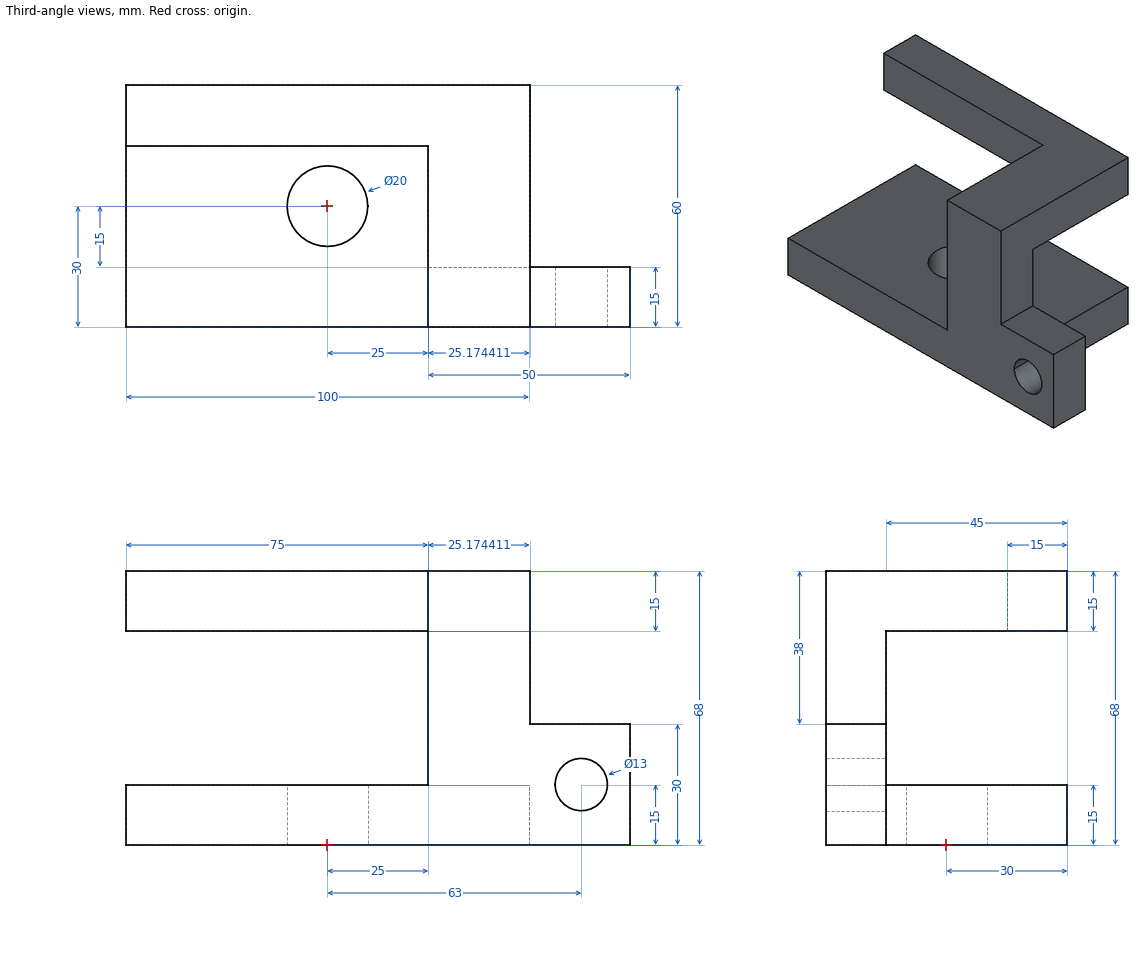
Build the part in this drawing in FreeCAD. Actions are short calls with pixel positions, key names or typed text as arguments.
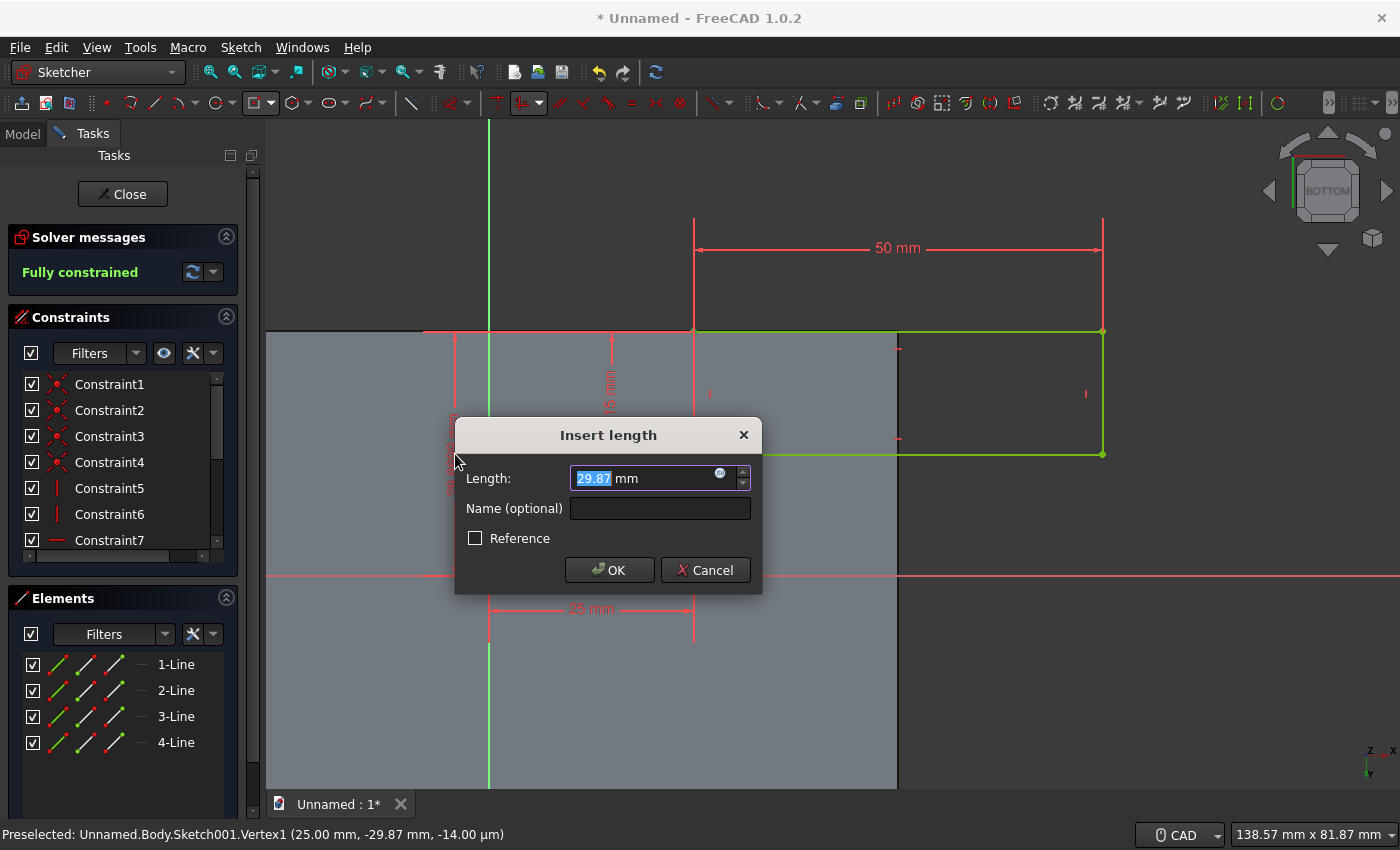
text(30)
key(Return)
key(Escape)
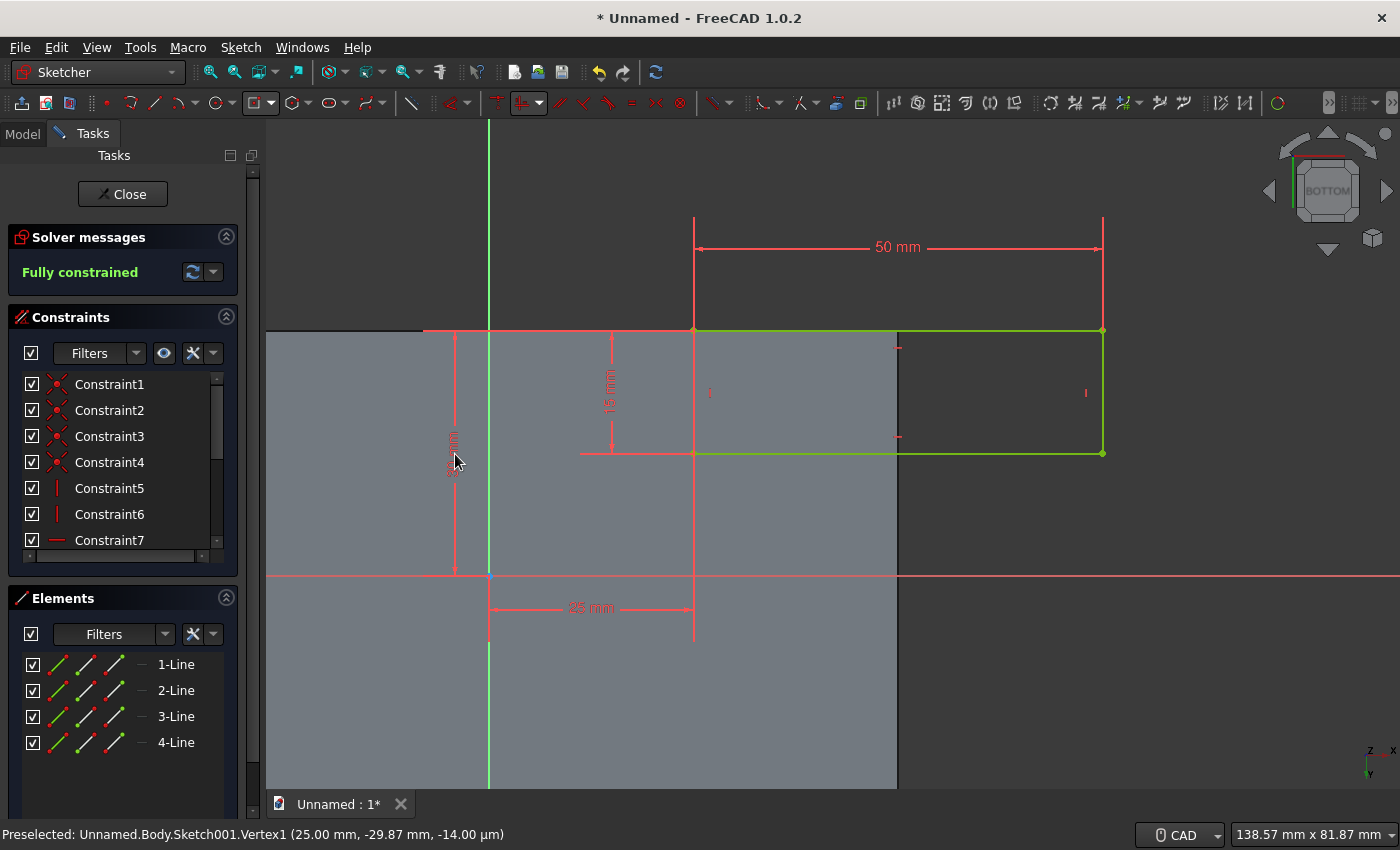
click(123, 194)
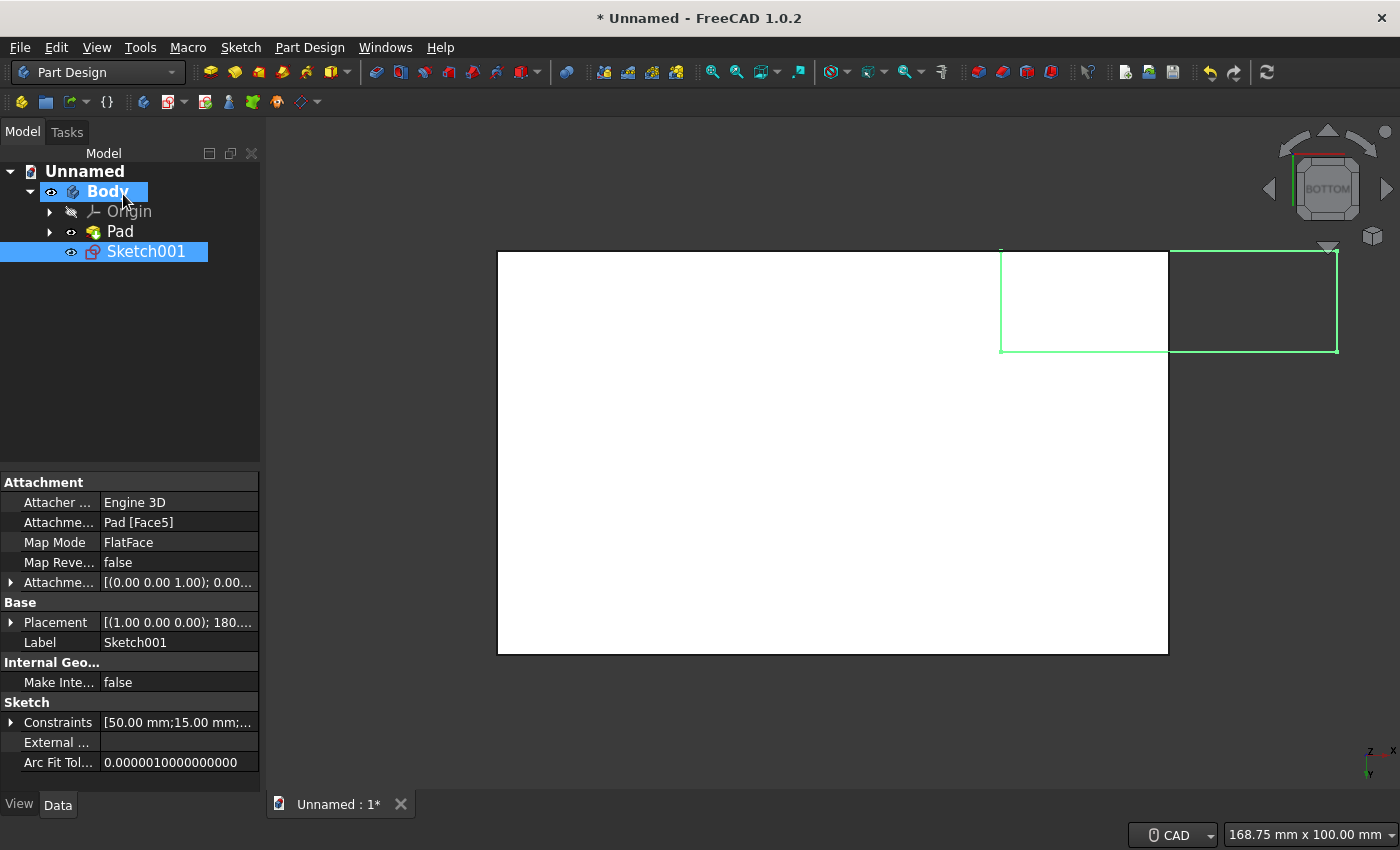
click(212, 72)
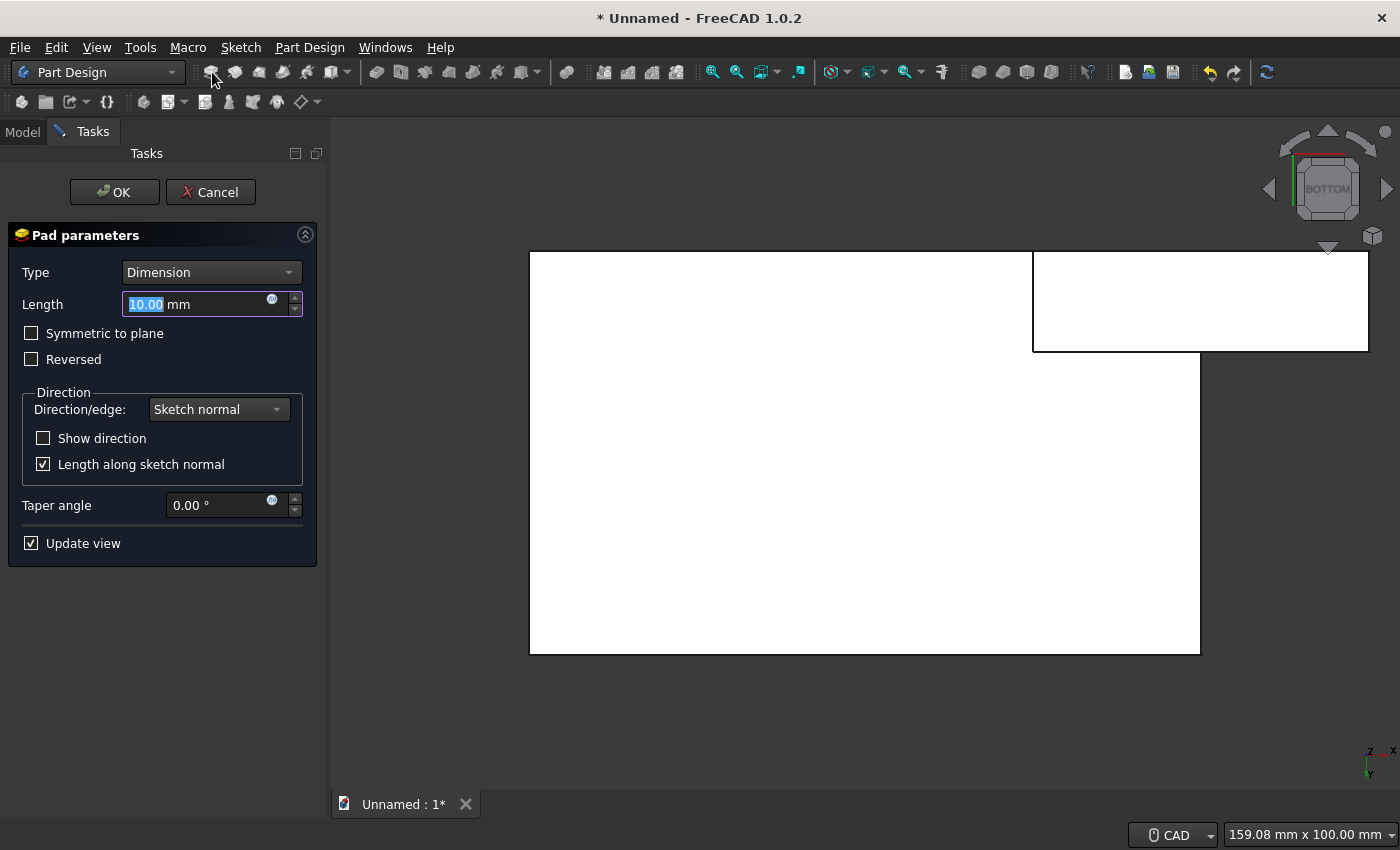
text(30)
key(Tab)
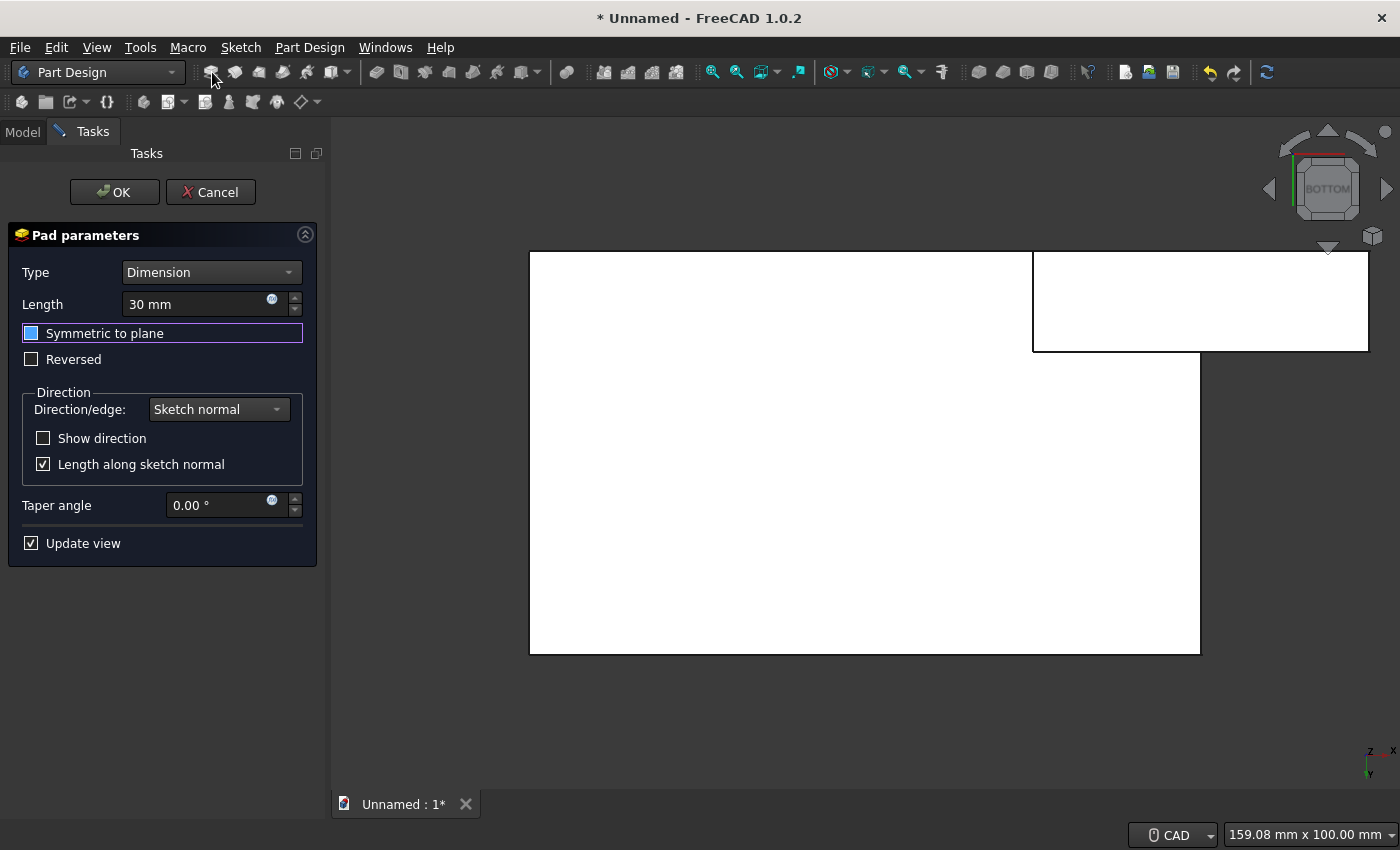
click(30, 359)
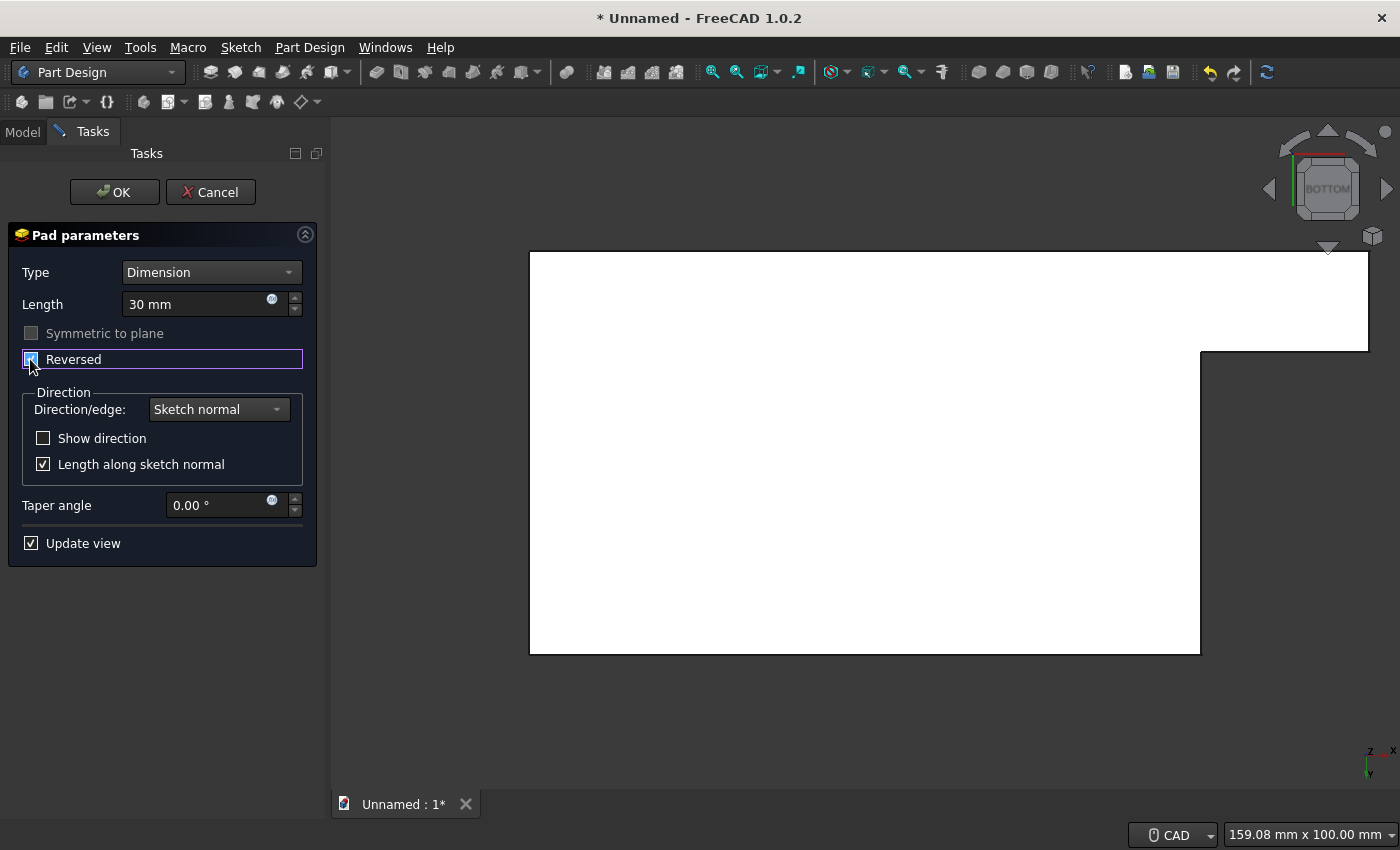
click(115, 192)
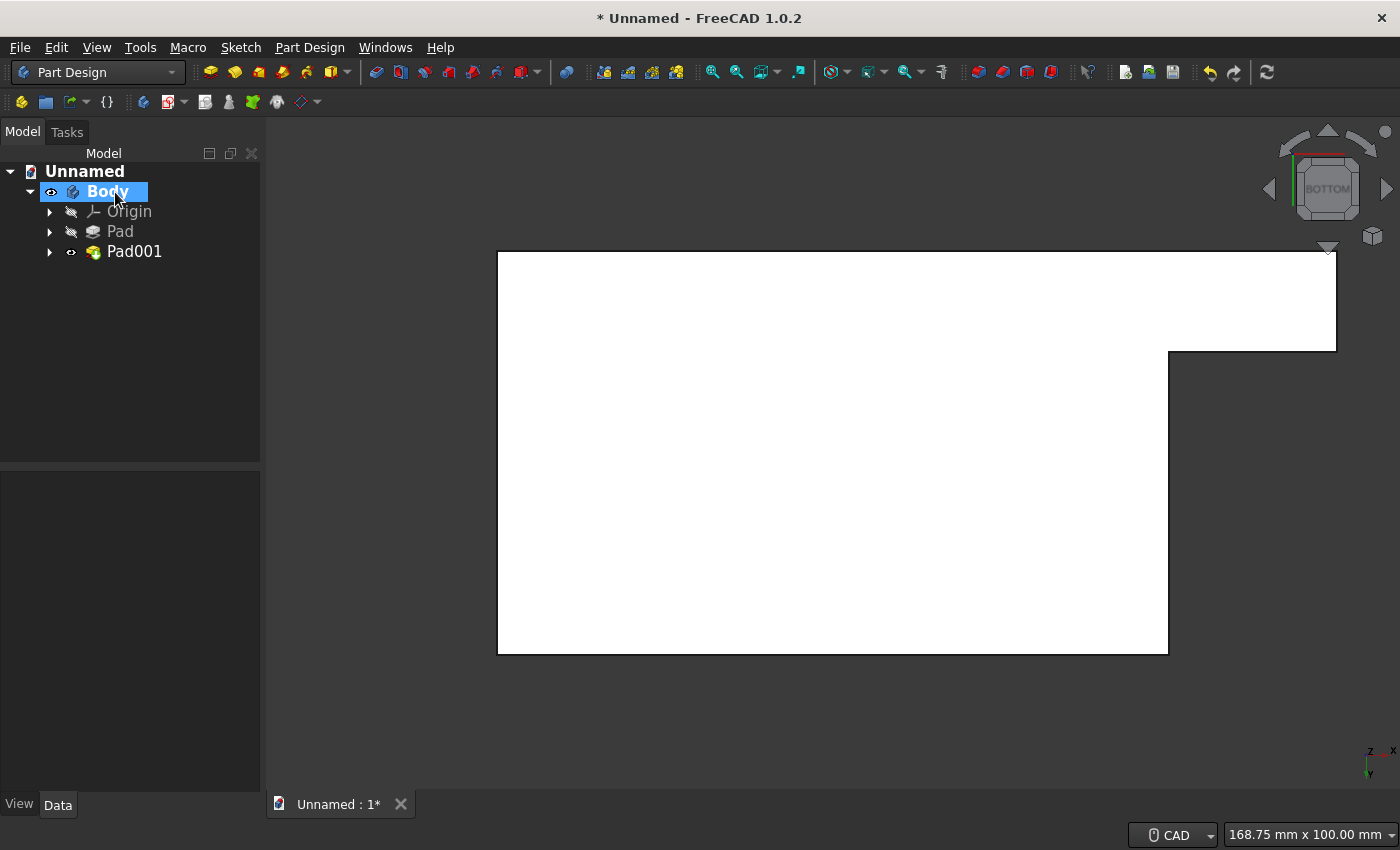
key(0)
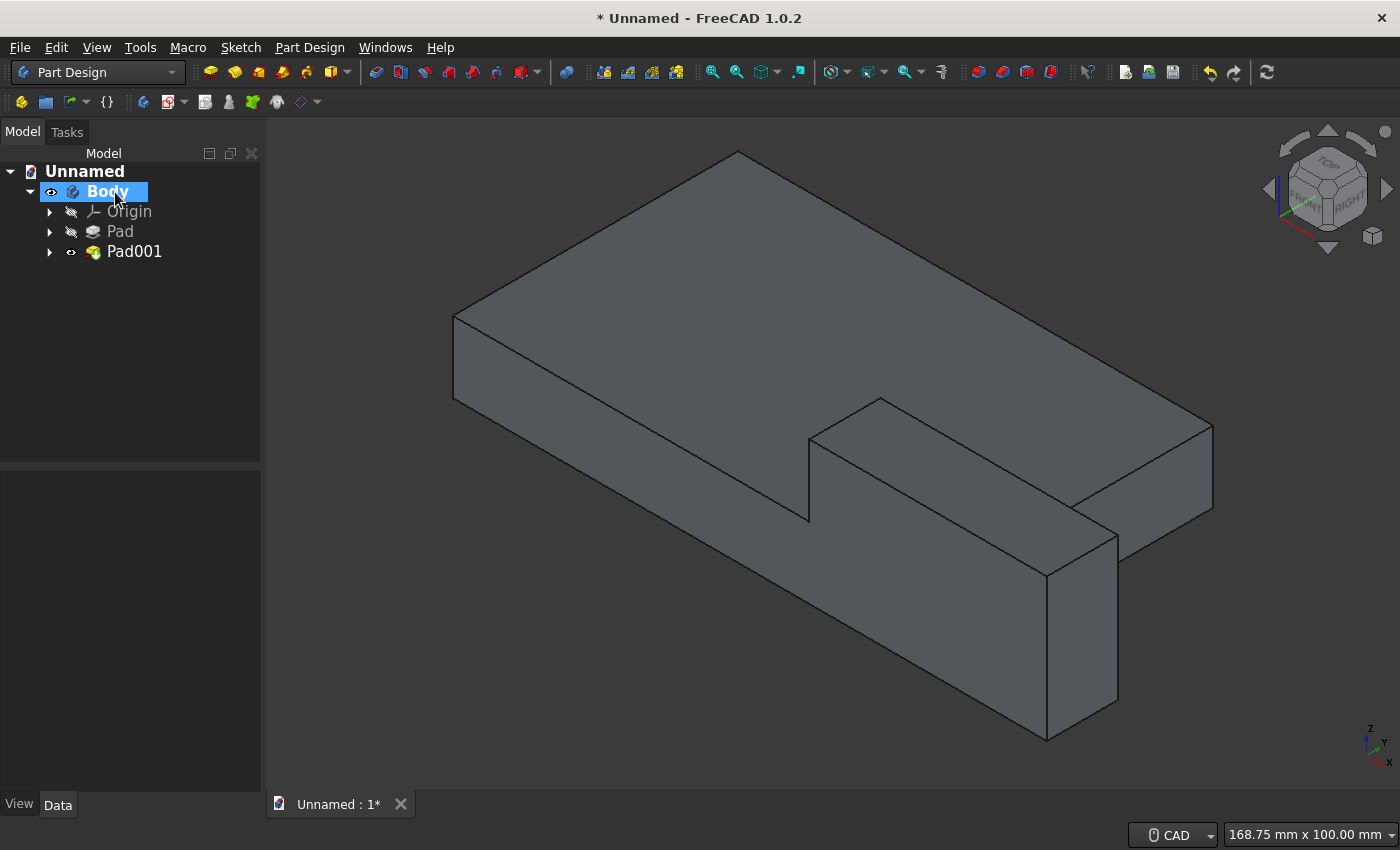
click(714, 72)